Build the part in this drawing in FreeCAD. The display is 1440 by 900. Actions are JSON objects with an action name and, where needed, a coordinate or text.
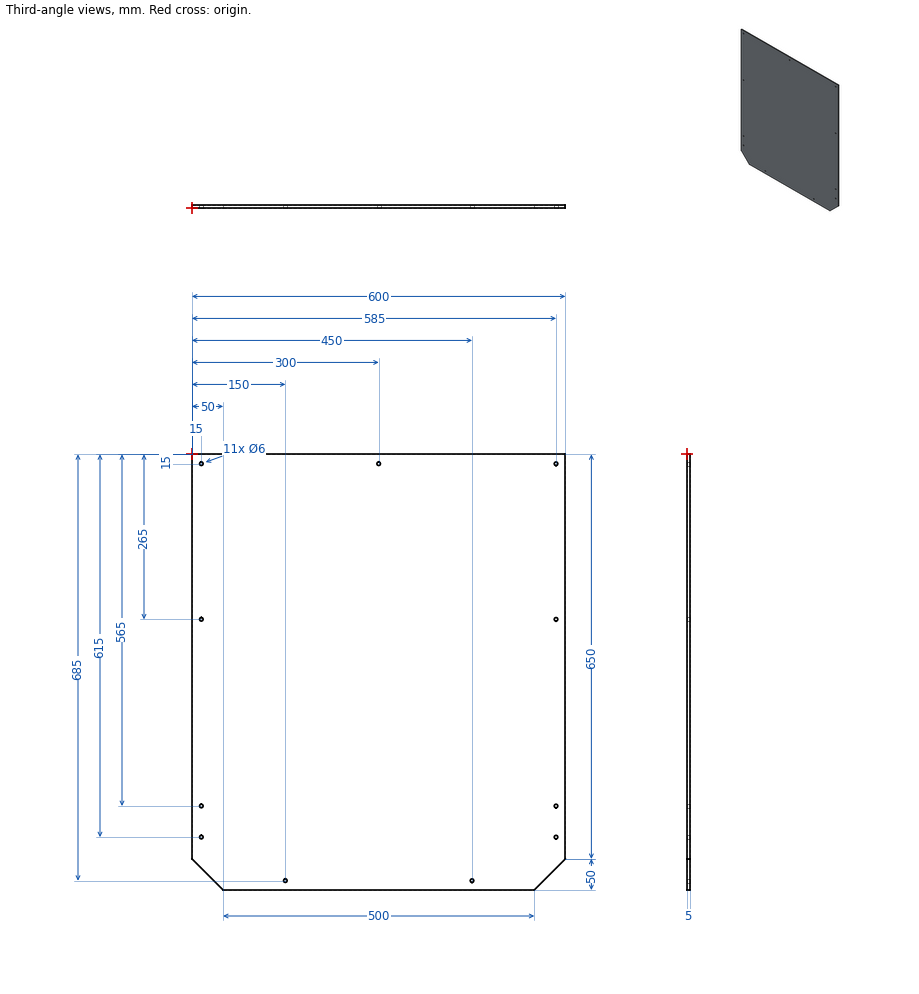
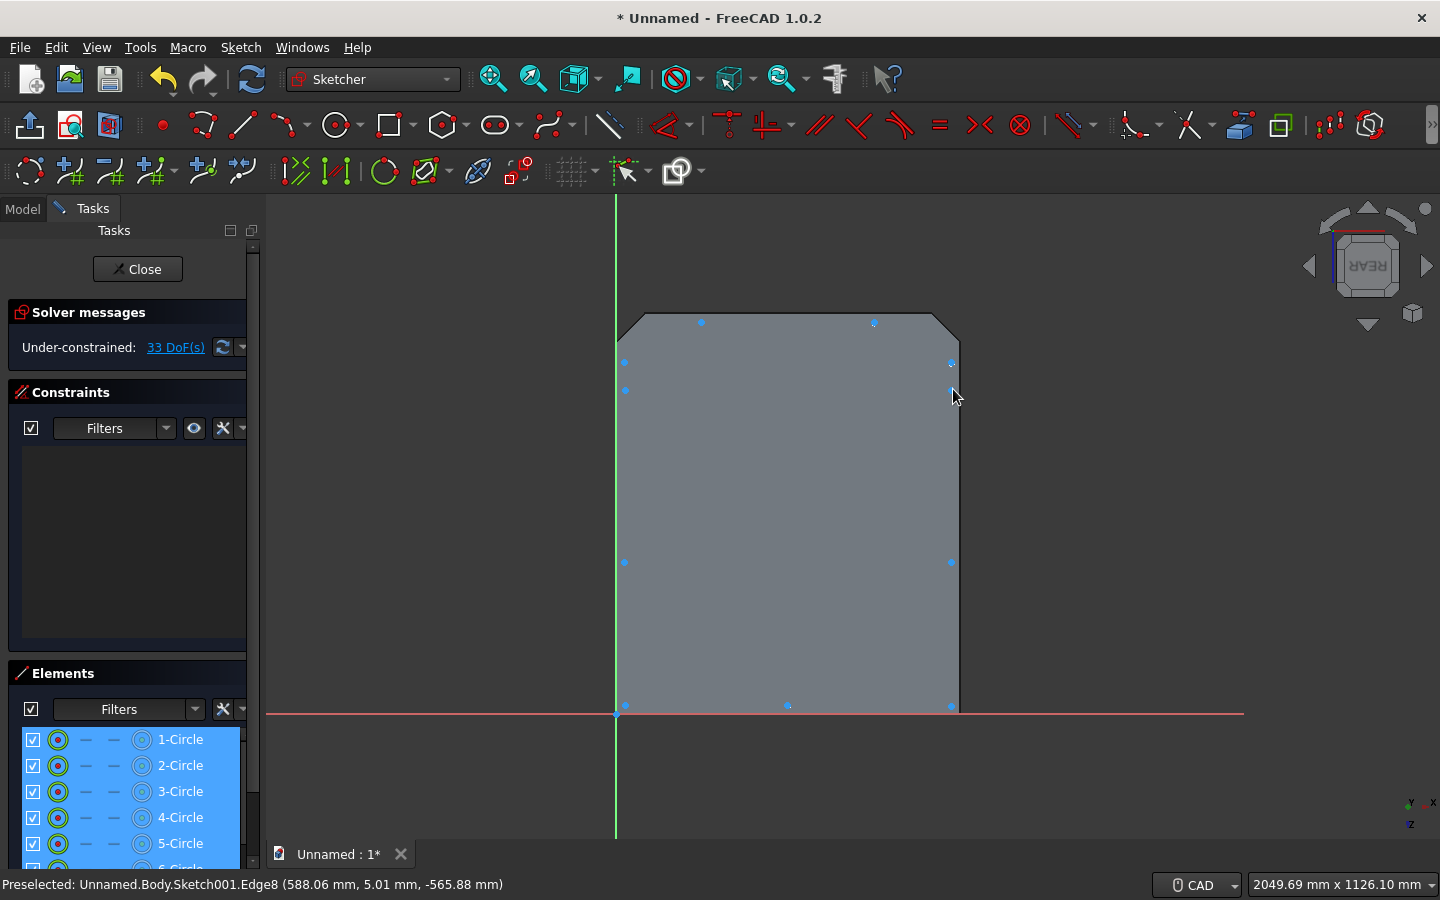
{"action": "scroll", "coordinate": [953, 361], "scroll_direction": "up", "scroll_amount": 9}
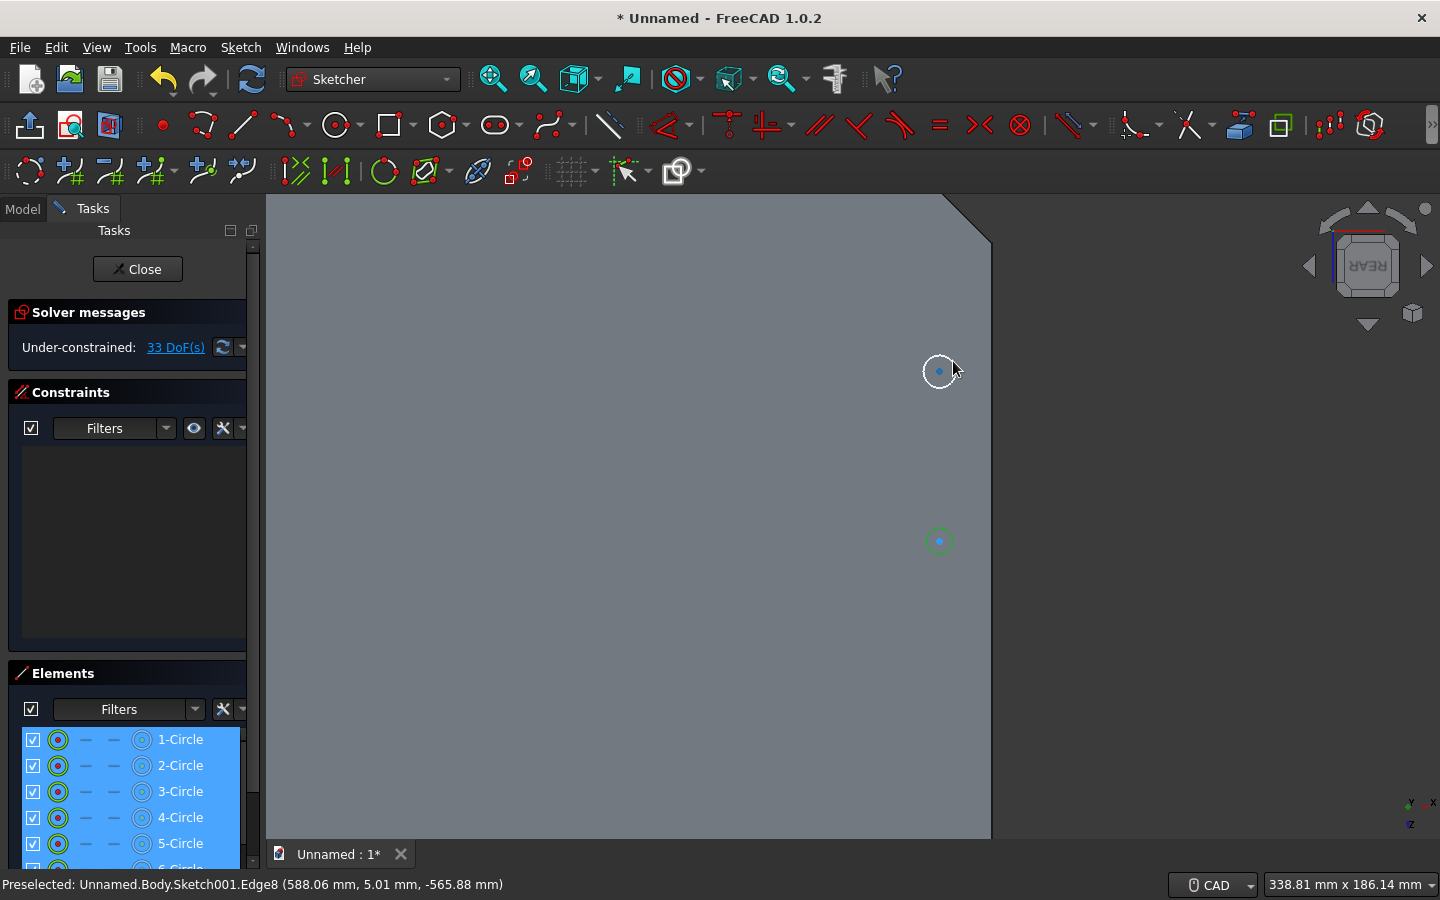
{"action": "left_click", "coordinate": [951, 360]}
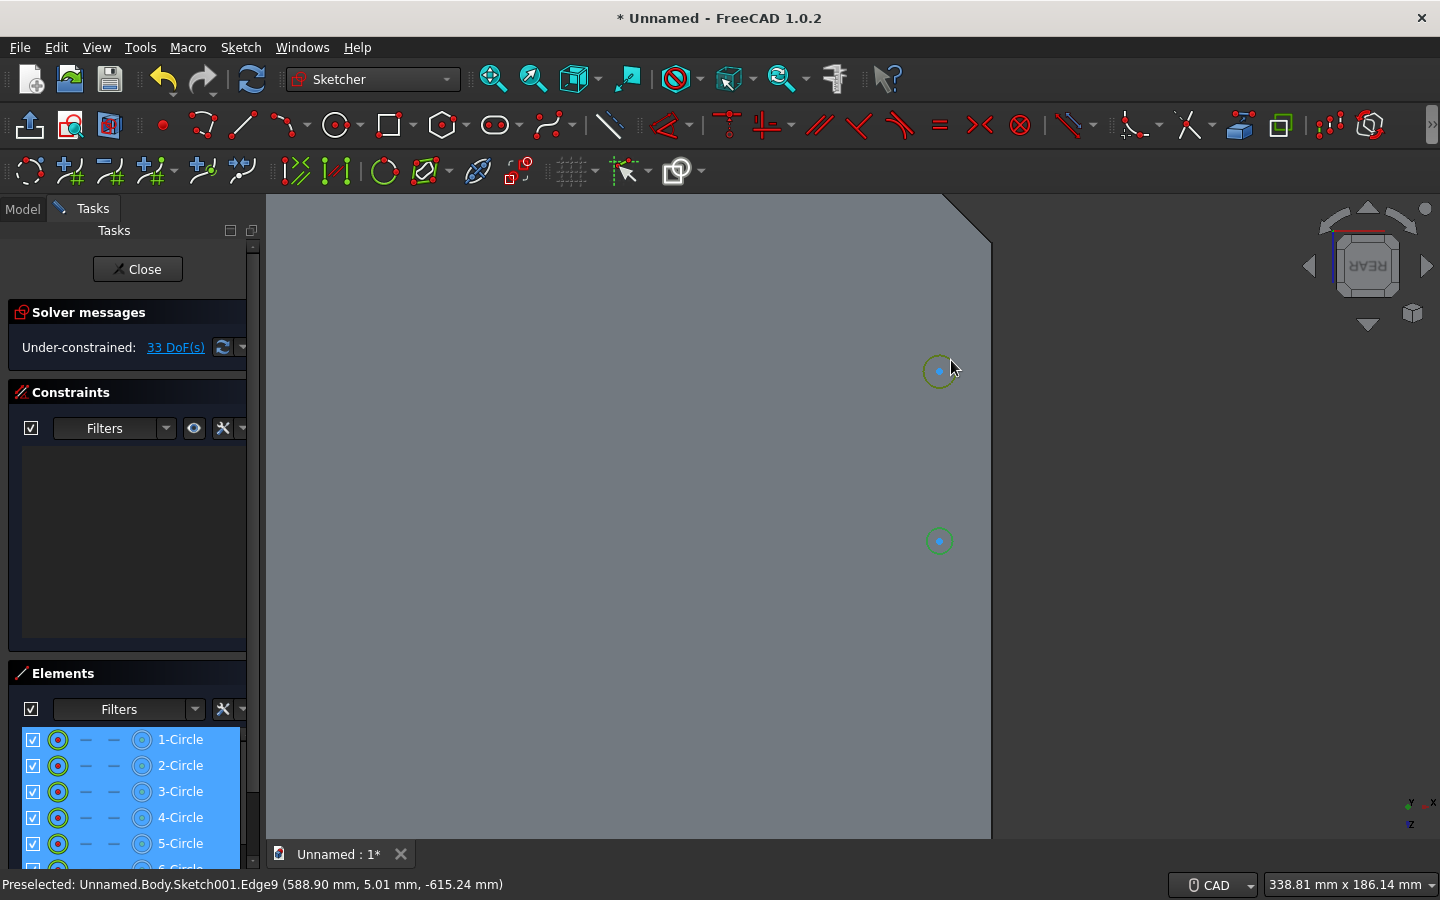
{"action": "scroll", "coordinate": [953, 361], "scroll_direction": "down", "scroll_amount": 9}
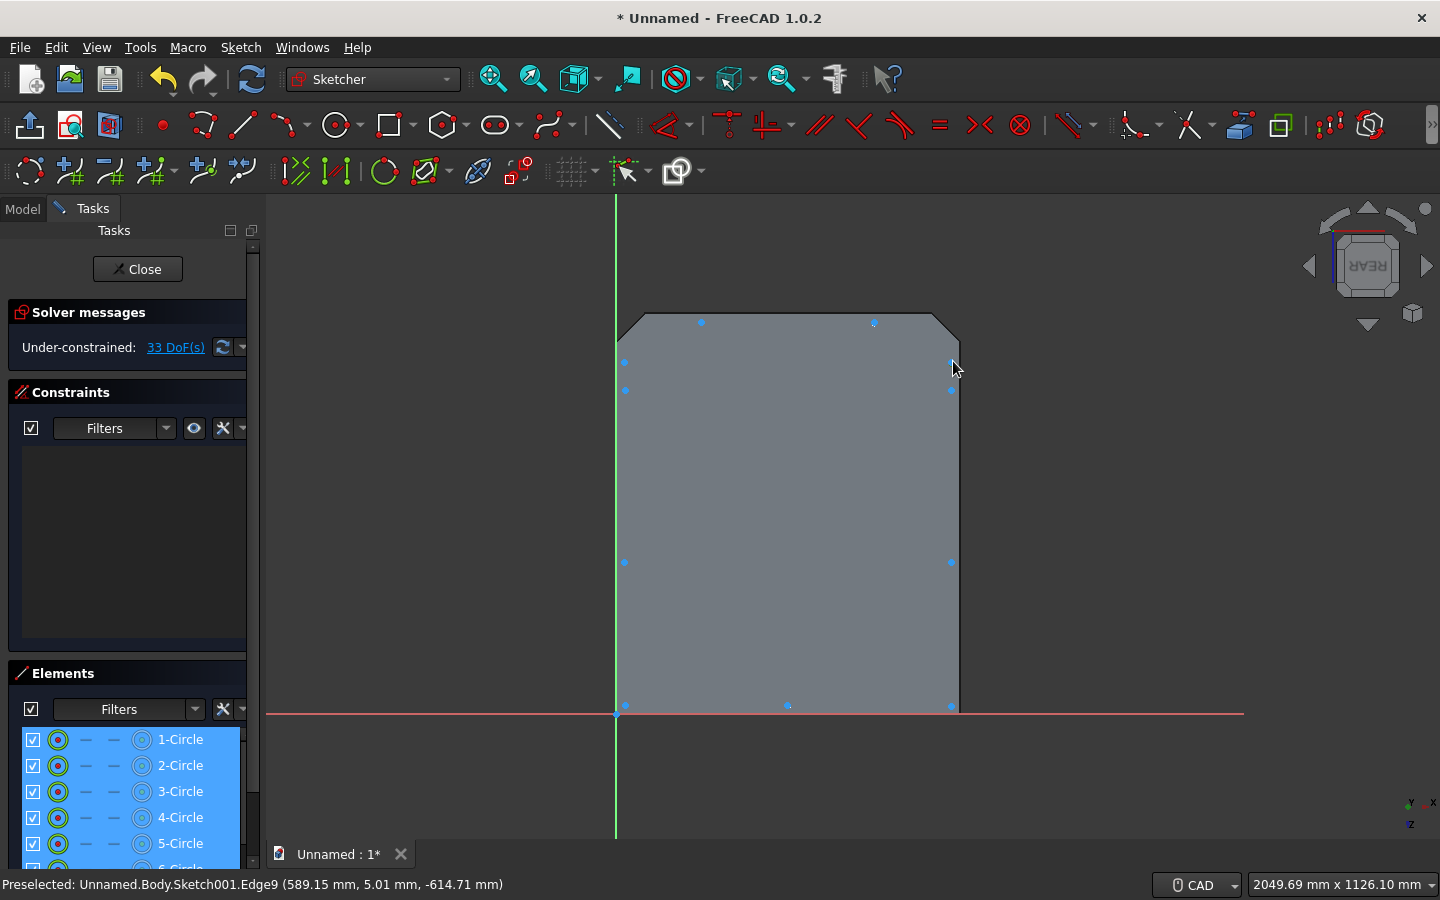
{"action": "scroll", "coordinate": [876, 321], "scroll_direction": "up", "scroll_amount": 9}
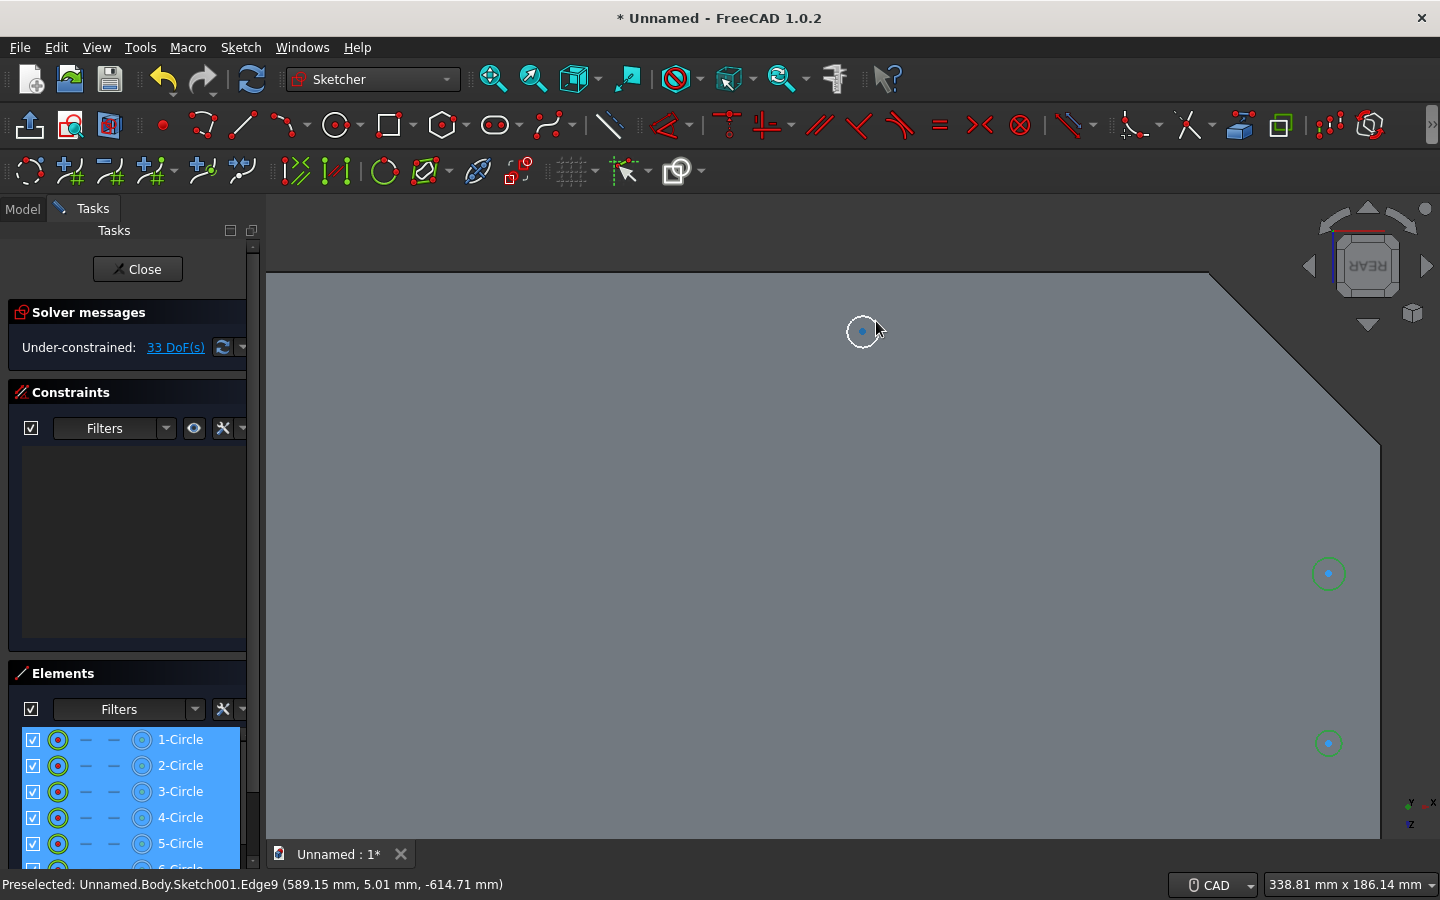
{"action": "left_click", "coordinate": [874, 321]}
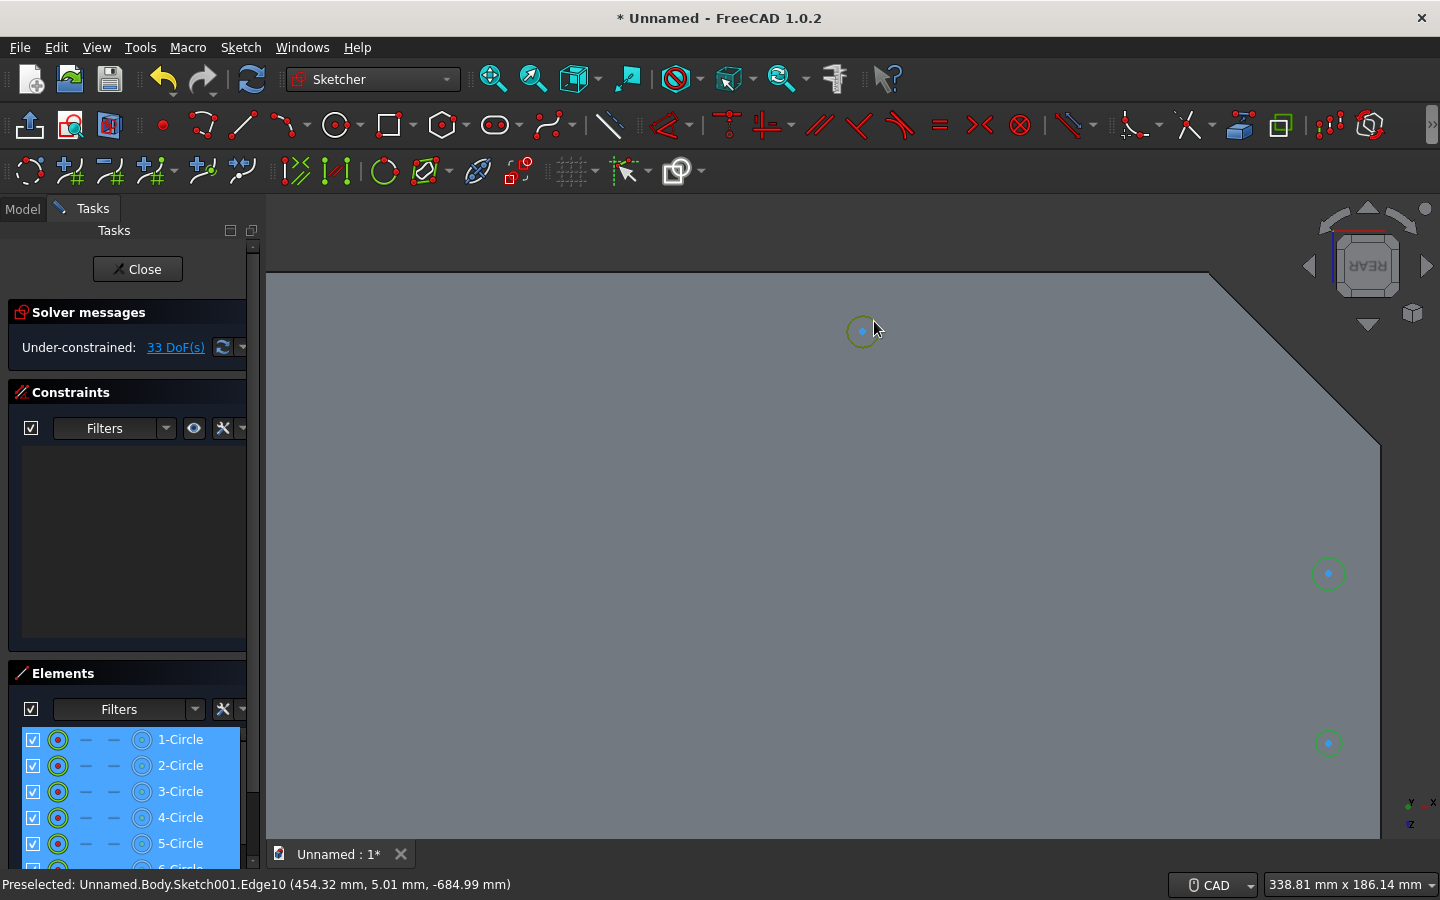
{"action": "scroll", "coordinate": [876, 321], "scroll_direction": "down", "scroll_amount": 9}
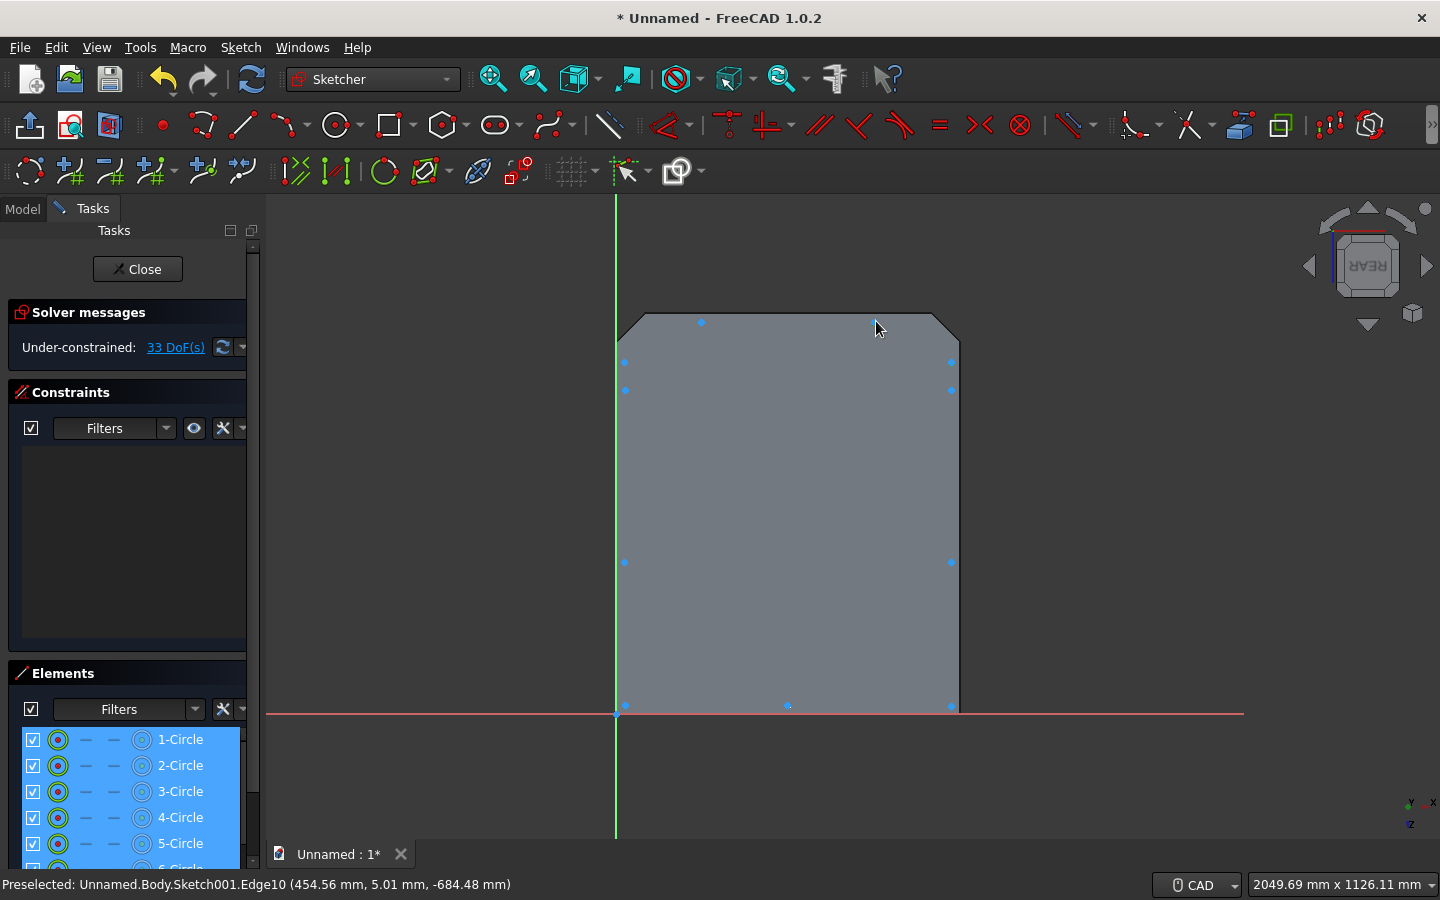
{"action": "scroll", "coordinate": [789, 704], "scroll_direction": "up", "scroll_amount": 10}